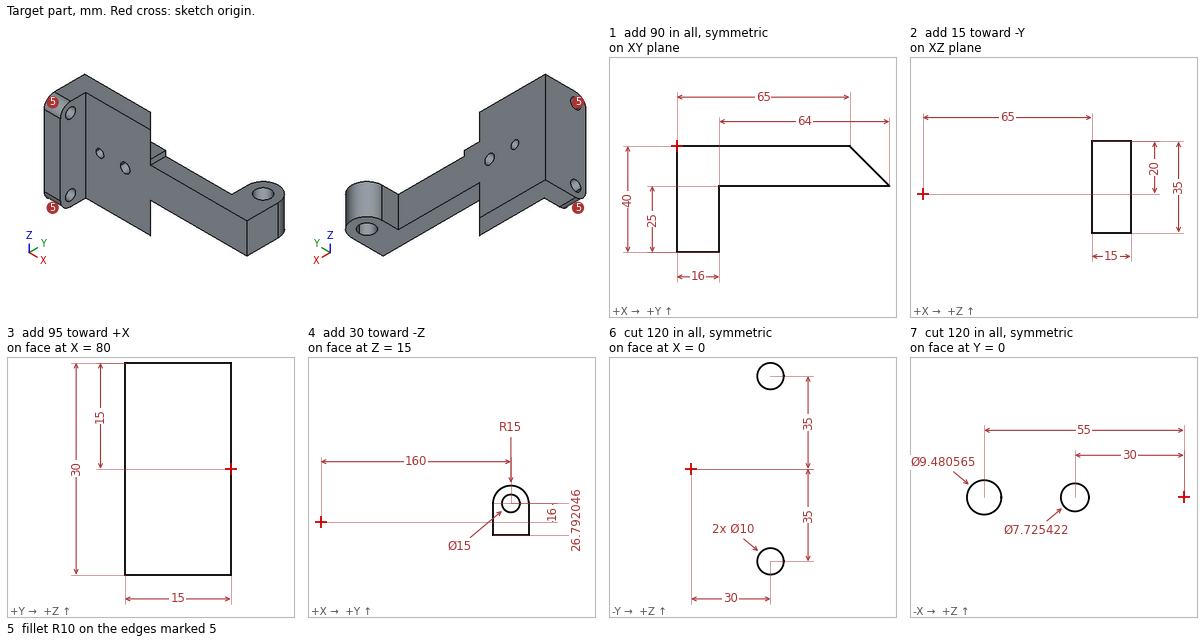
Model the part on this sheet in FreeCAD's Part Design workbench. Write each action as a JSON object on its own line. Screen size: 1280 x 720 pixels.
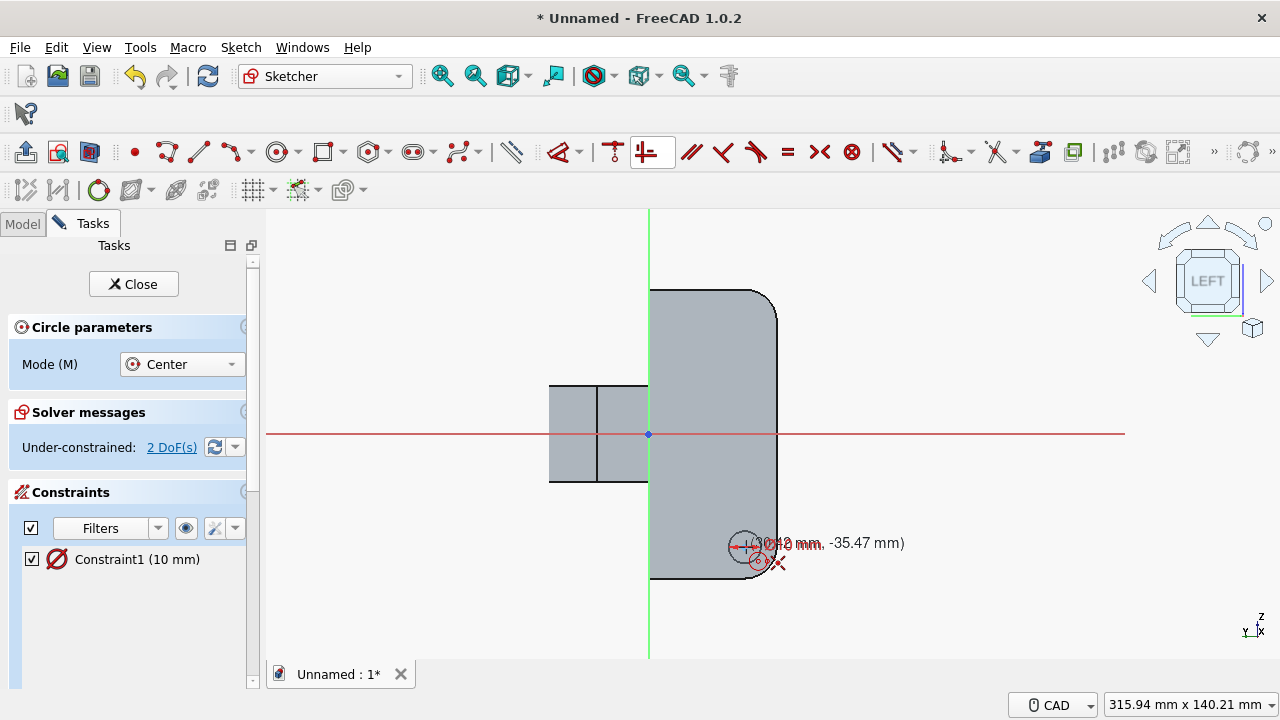
{"action": "scroll", "coordinate": [745, 322], "scroll_direction": "up", "scroll_amount": 2}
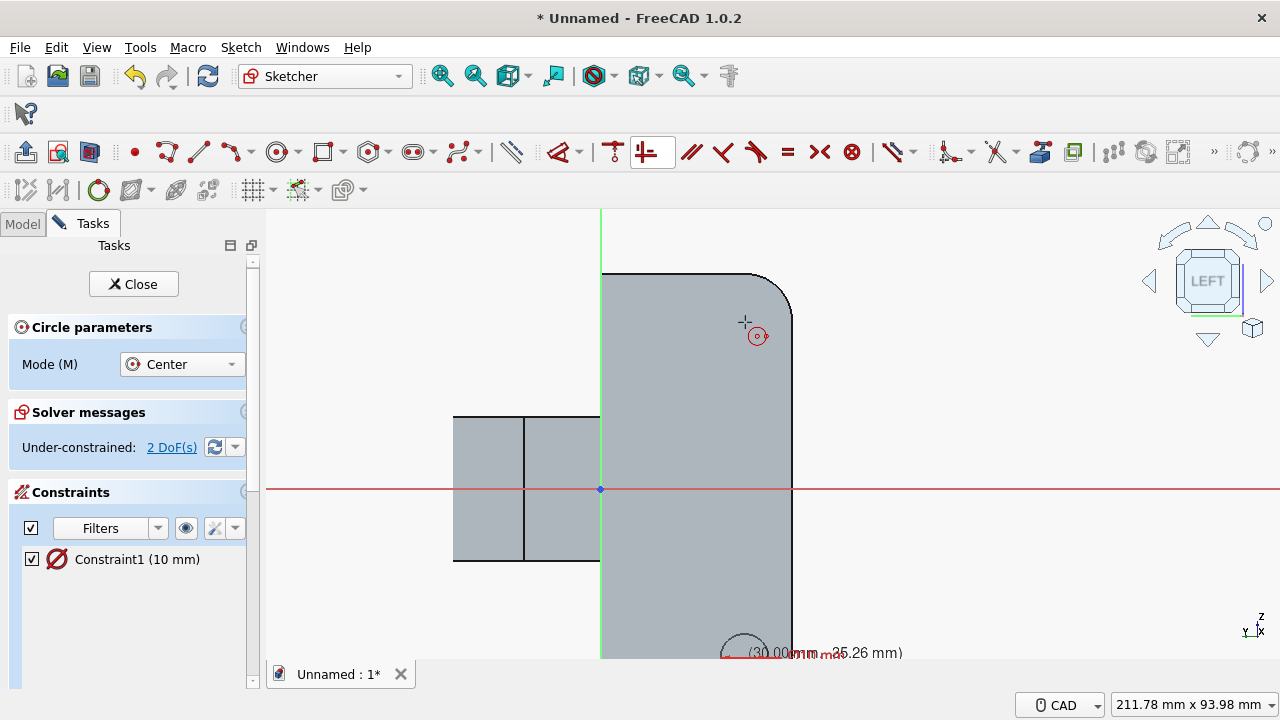
{"action": "left_click", "coordinate": [744, 322]}
{"action": "mouse_move", "coordinate": [761, 305]}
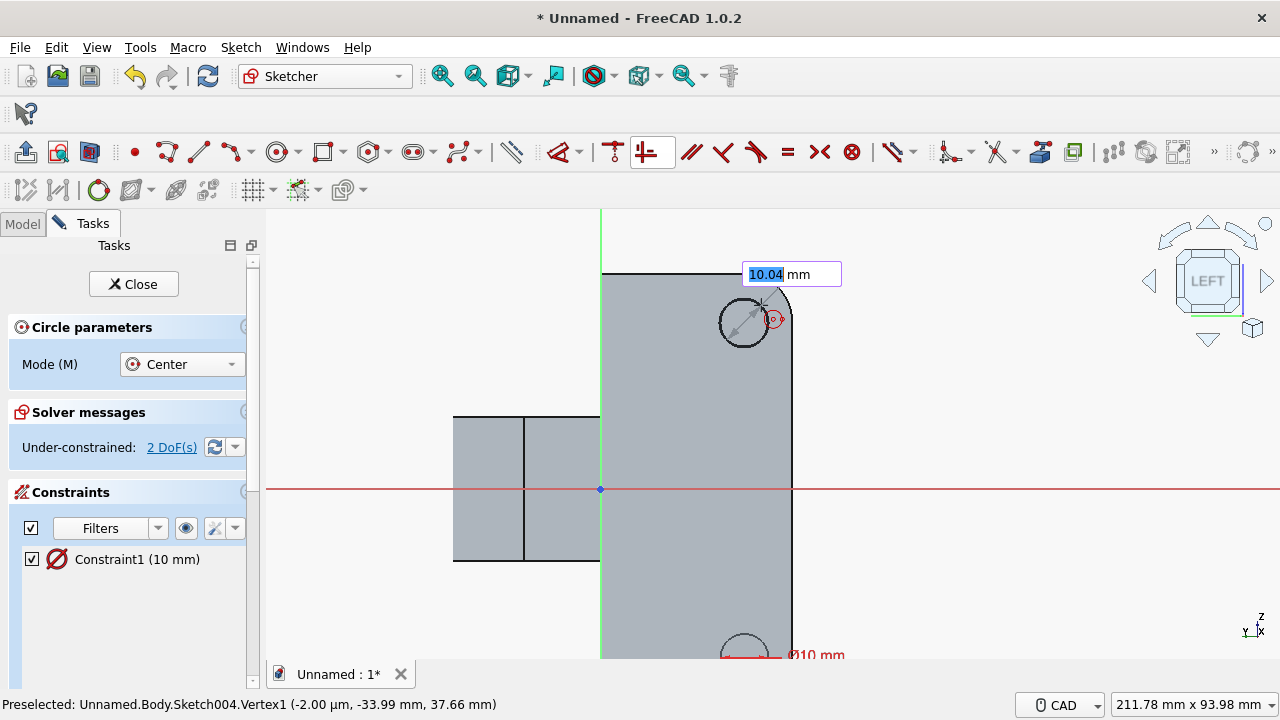
{"action": "type", "text": "10"}
{"action": "key", "text": "Return"}
{"action": "key", "text": "Escape"}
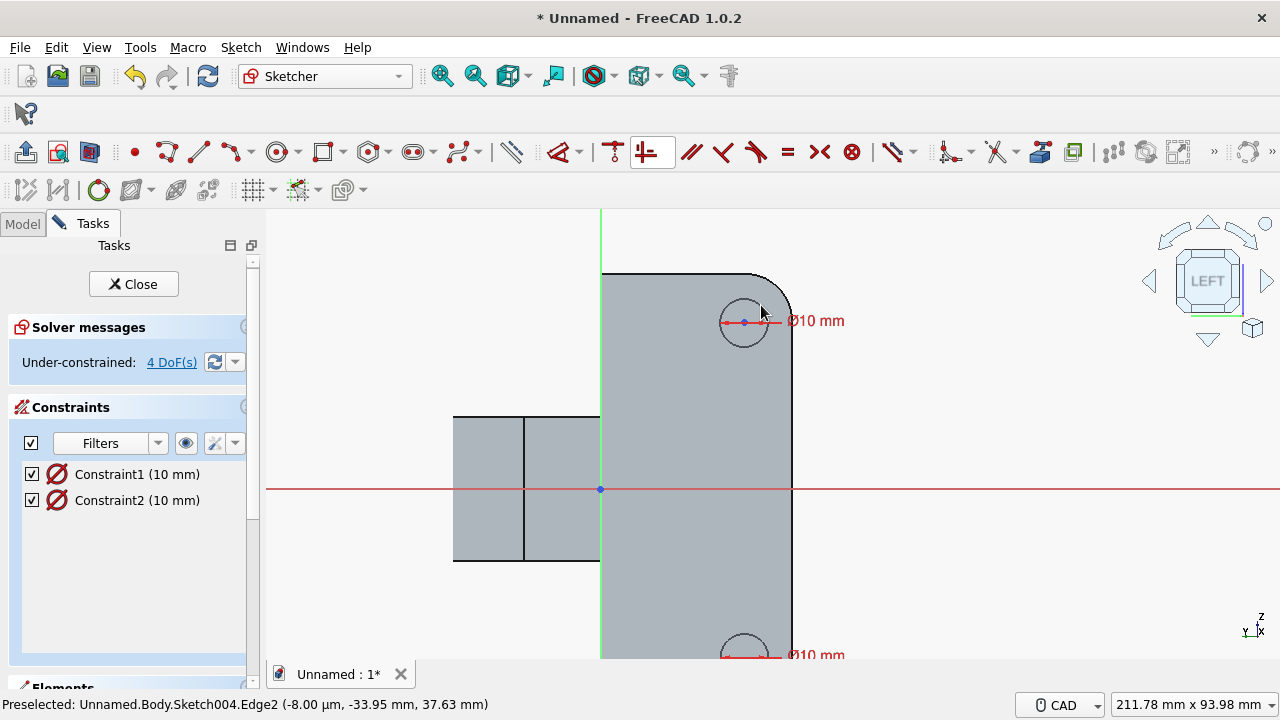
{"action": "scroll", "coordinate": [745, 322], "scroll_direction": "down", "scroll_amount": 2}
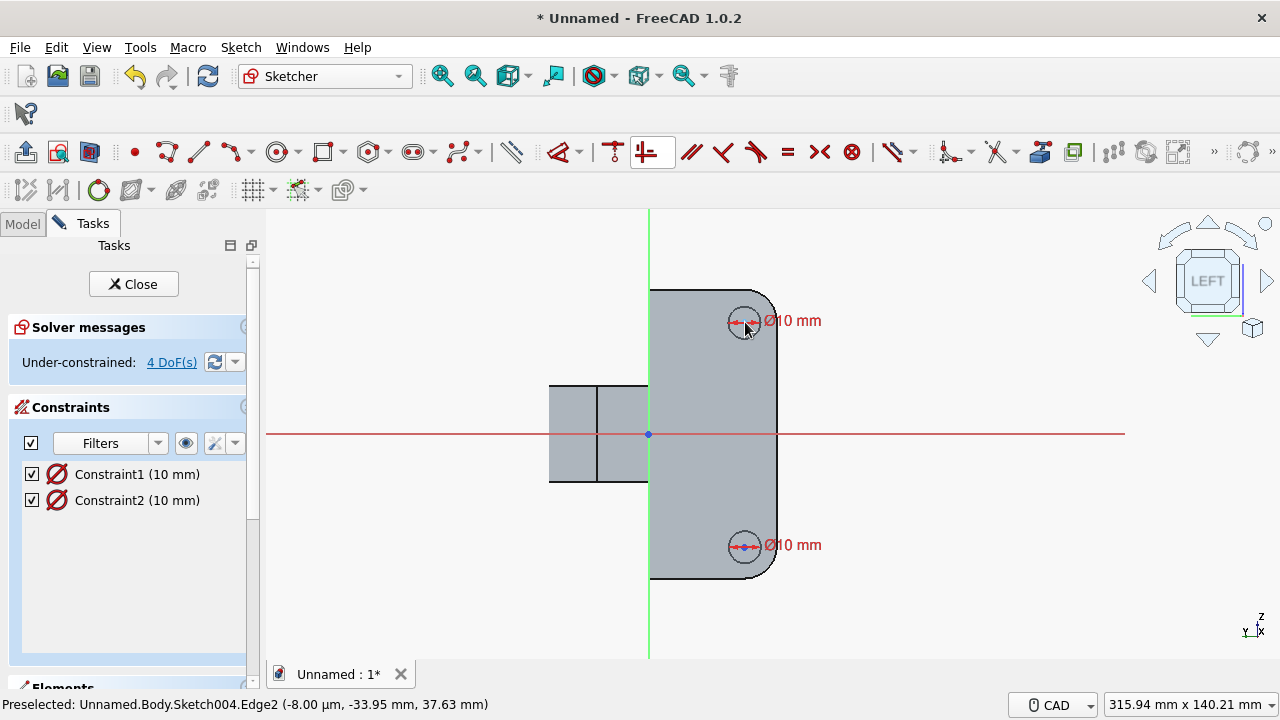
{"action": "left_click", "coordinate": [745, 547]}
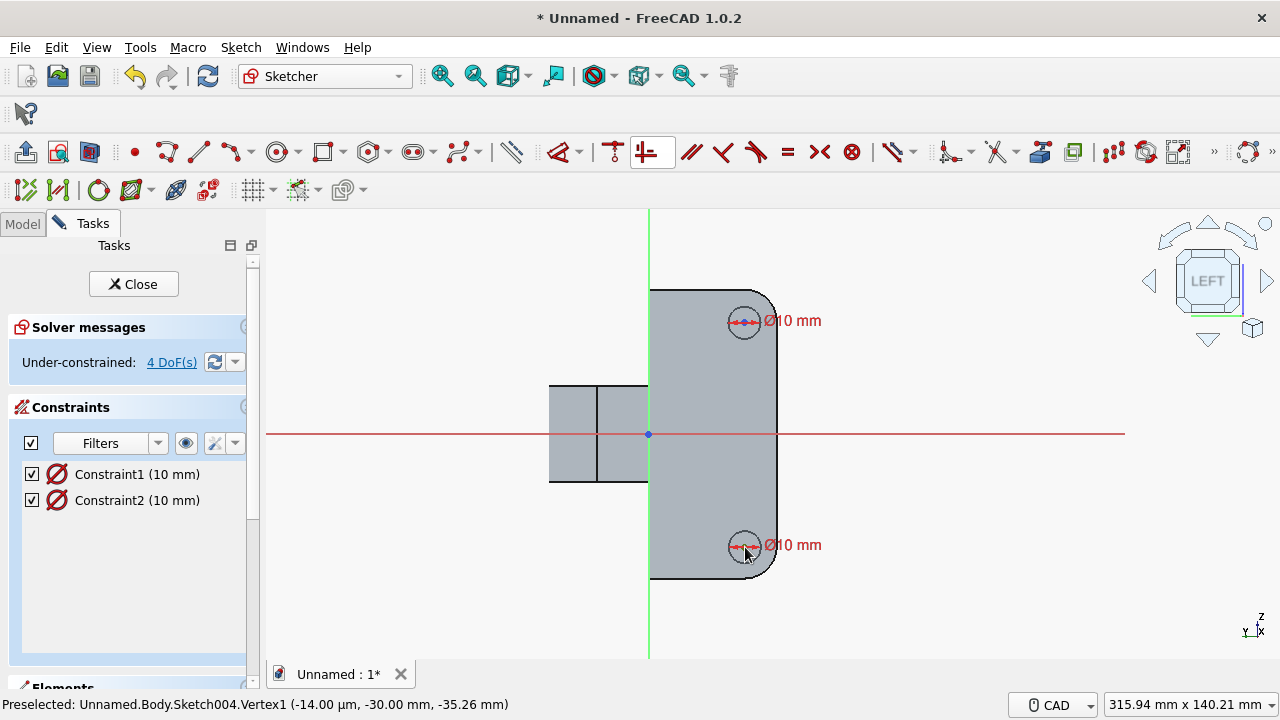
{"action": "left_click", "coordinate": [744, 323]}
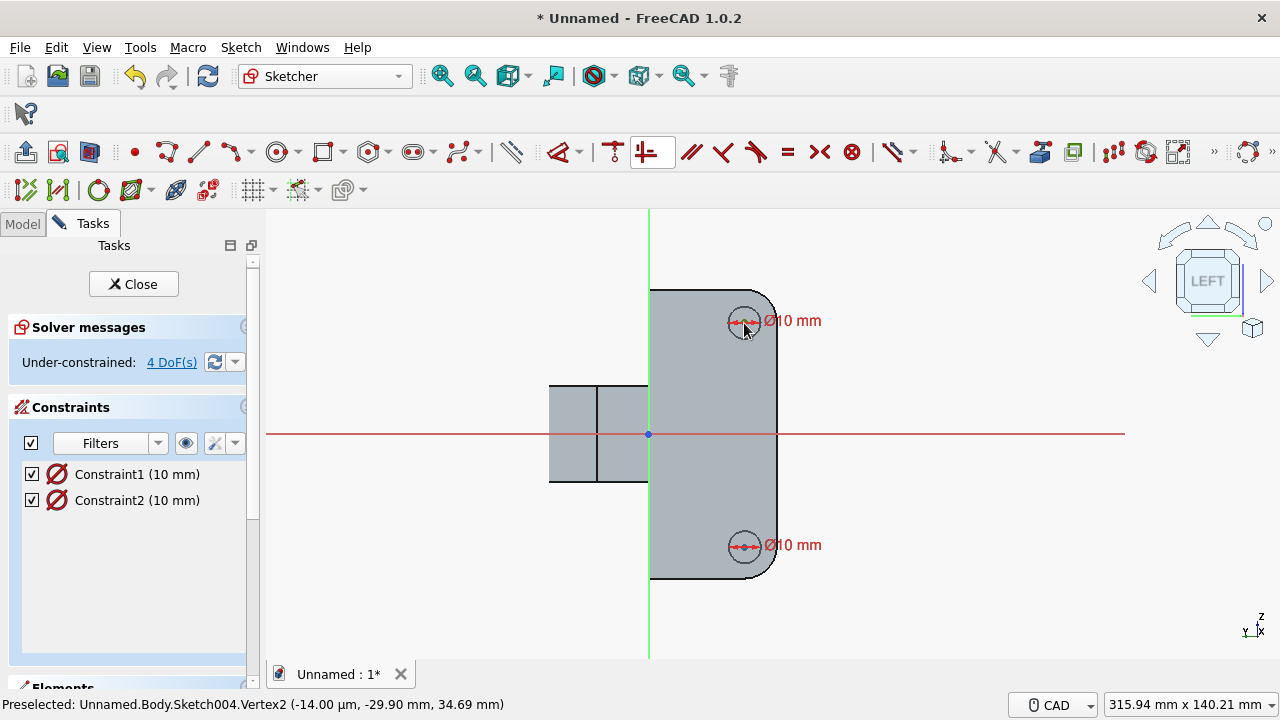
{"action": "key", "text": "v"}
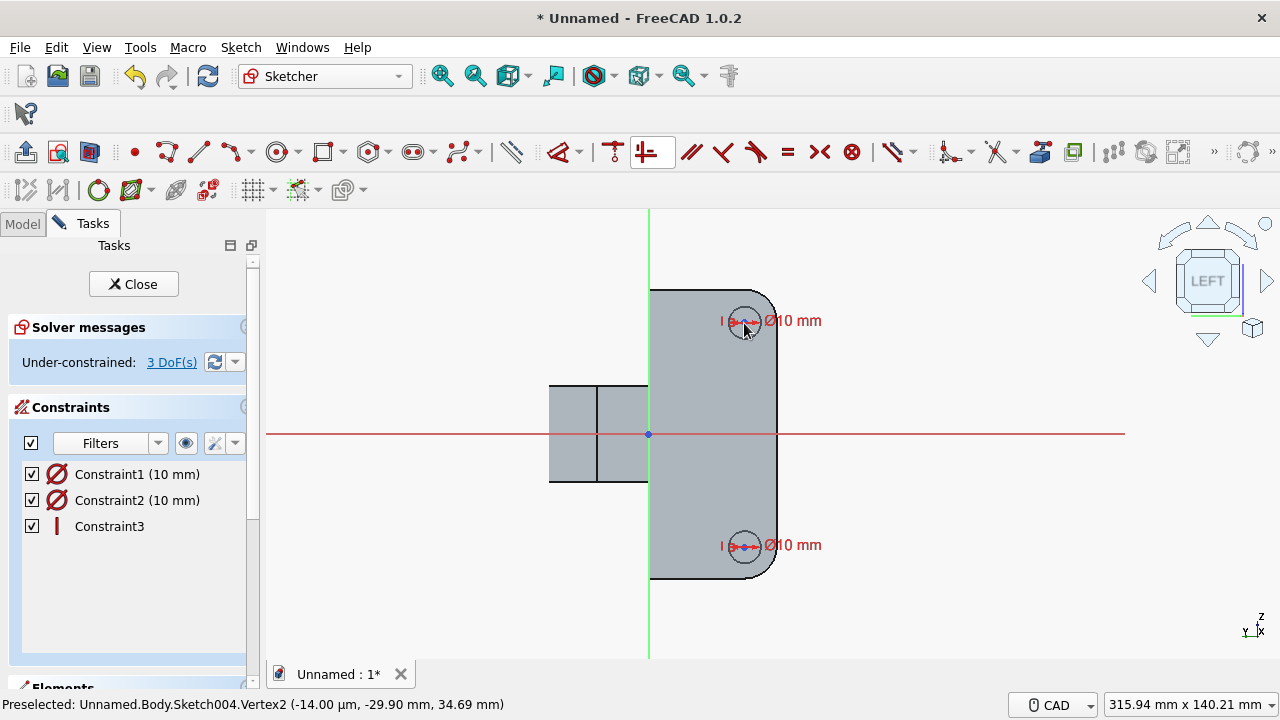
{"action": "left_click", "coordinate": [558, 152]}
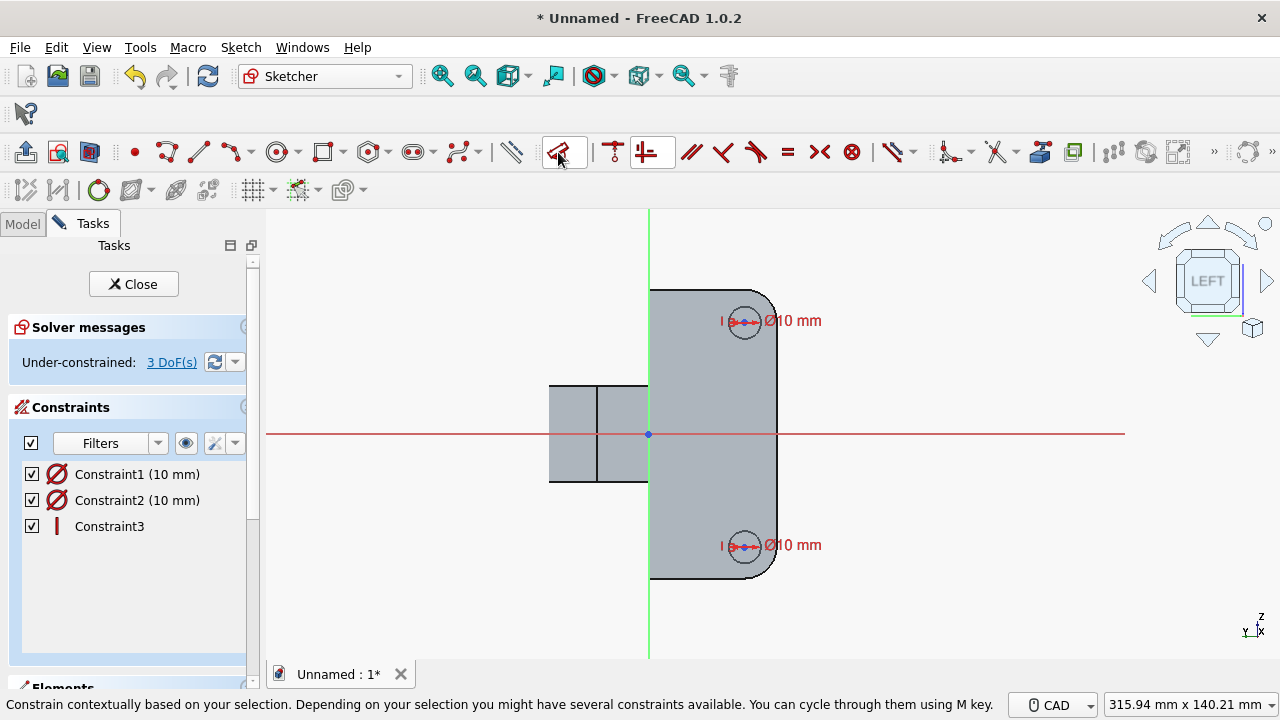
{"action": "left_click", "coordinate": [745, 547]}
{"action": "left_click", "coordinate": [697, 581]}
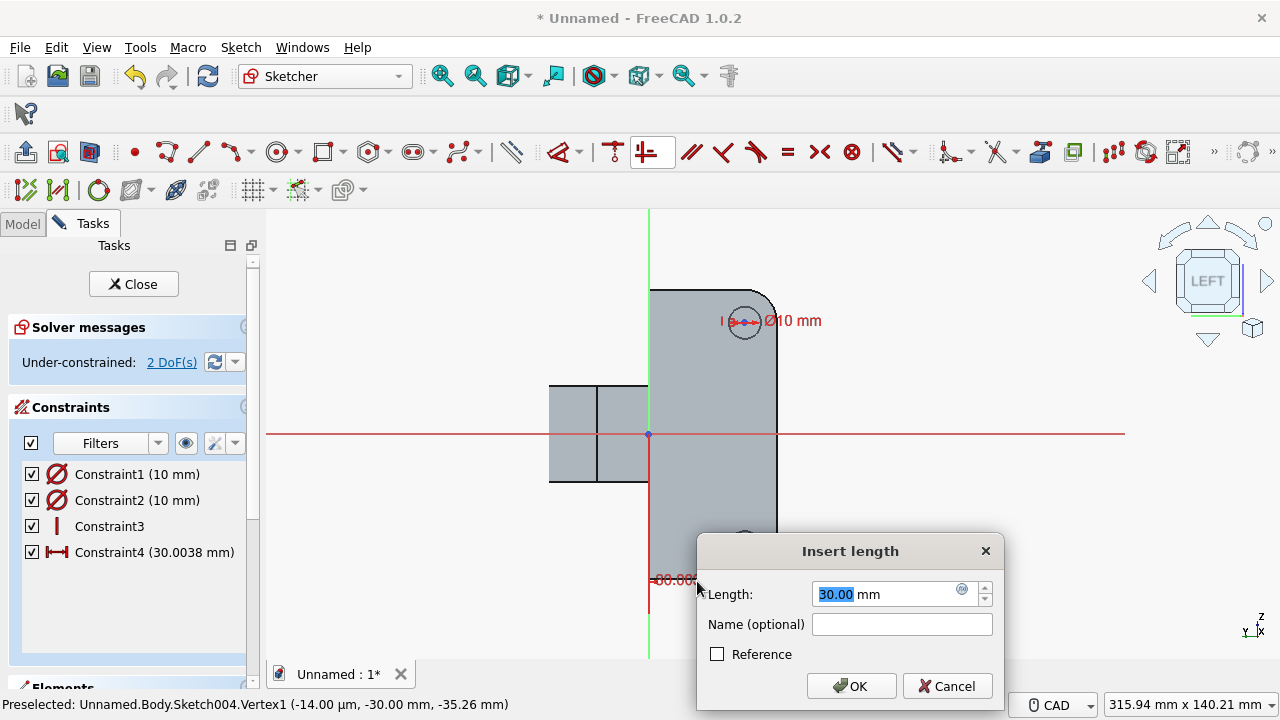
{"action": "type", "text": "30"}
{"action": "key", "text": "Return"}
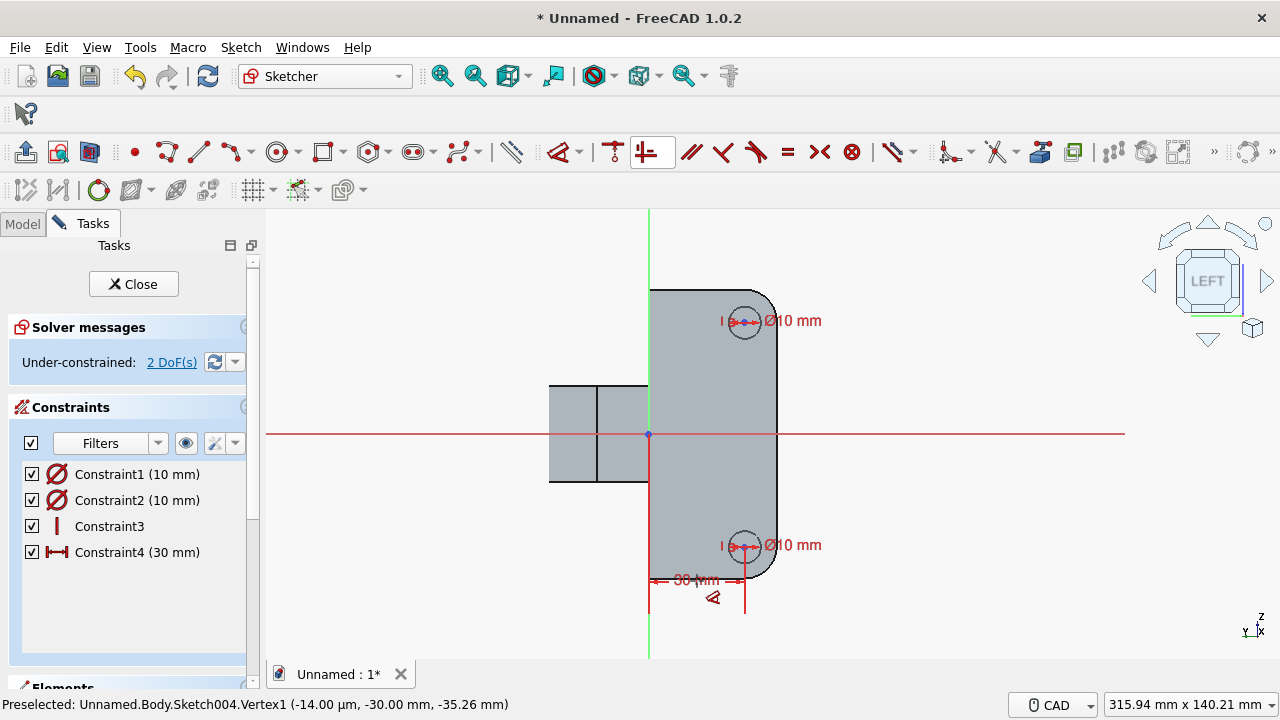
{"action": "left_click", "coordinate": [745, 547]}
{"action": "left_click", "coordinate": [615, 491]}